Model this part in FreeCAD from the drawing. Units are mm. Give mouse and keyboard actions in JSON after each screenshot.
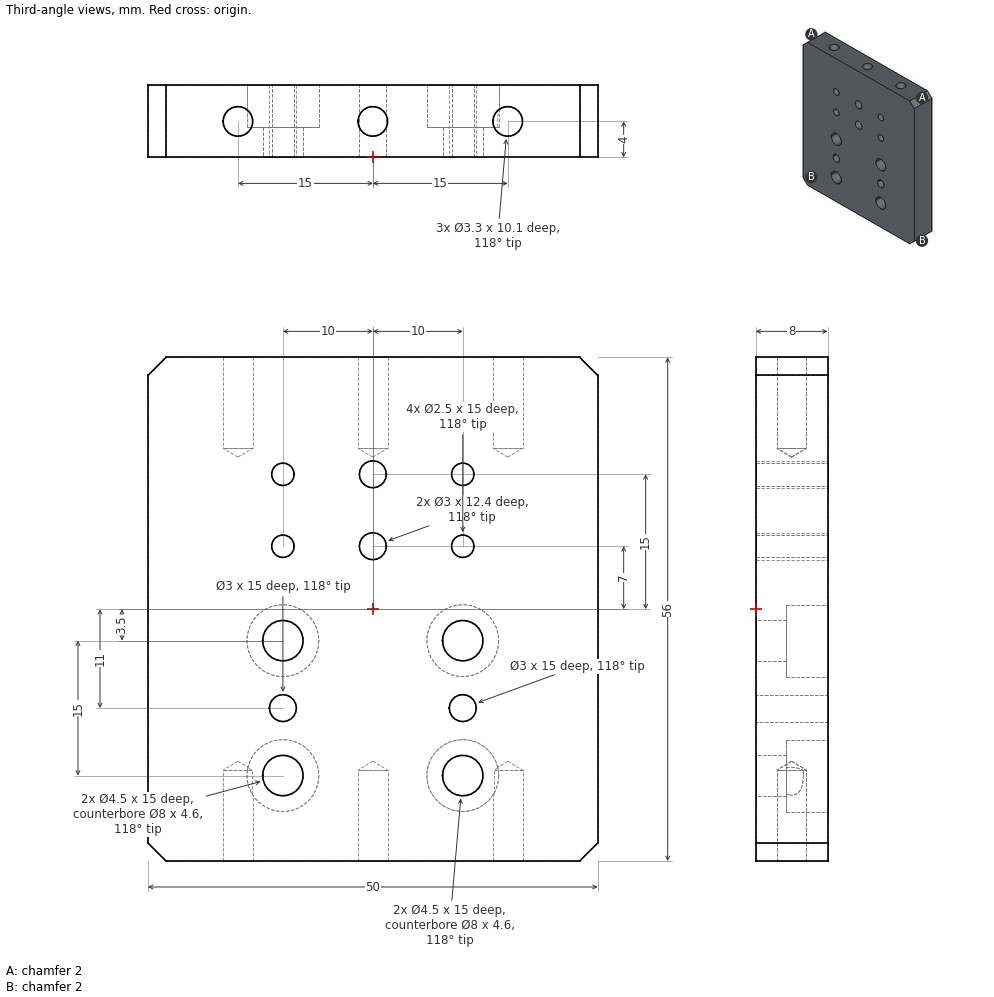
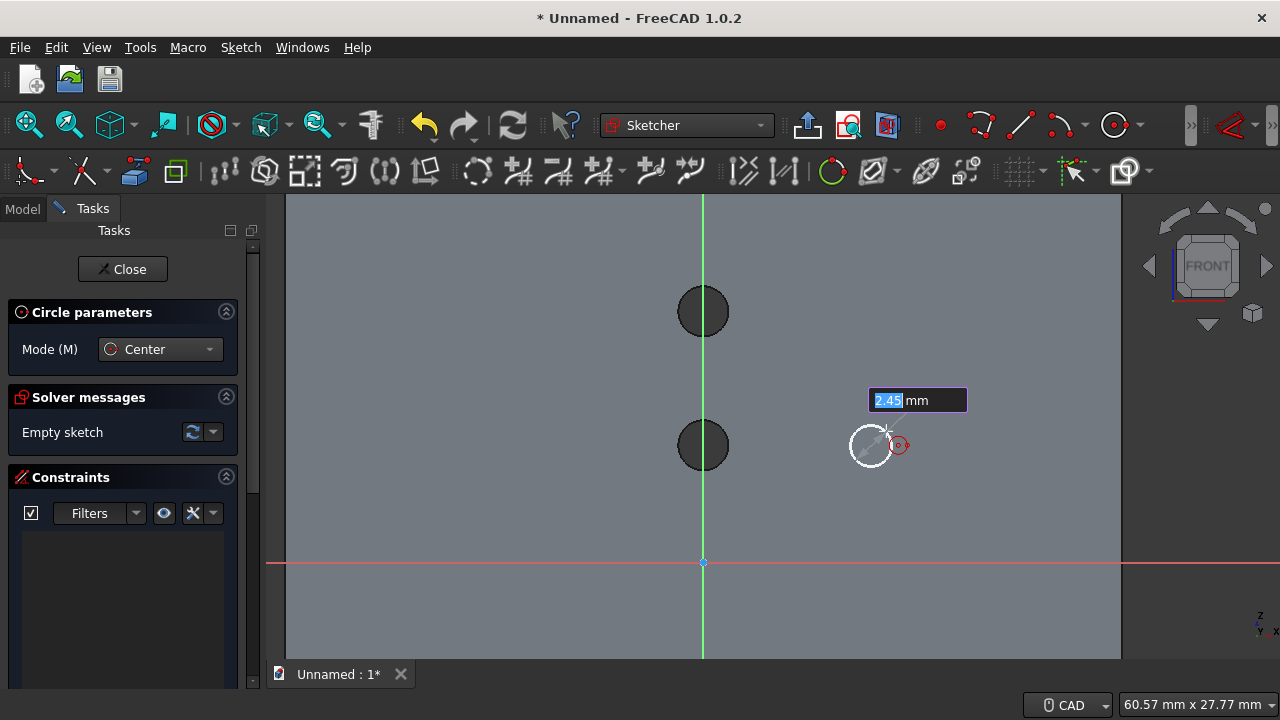
{"action": "type", "text": "2.5"}
{"action": "key", "text": "Return"}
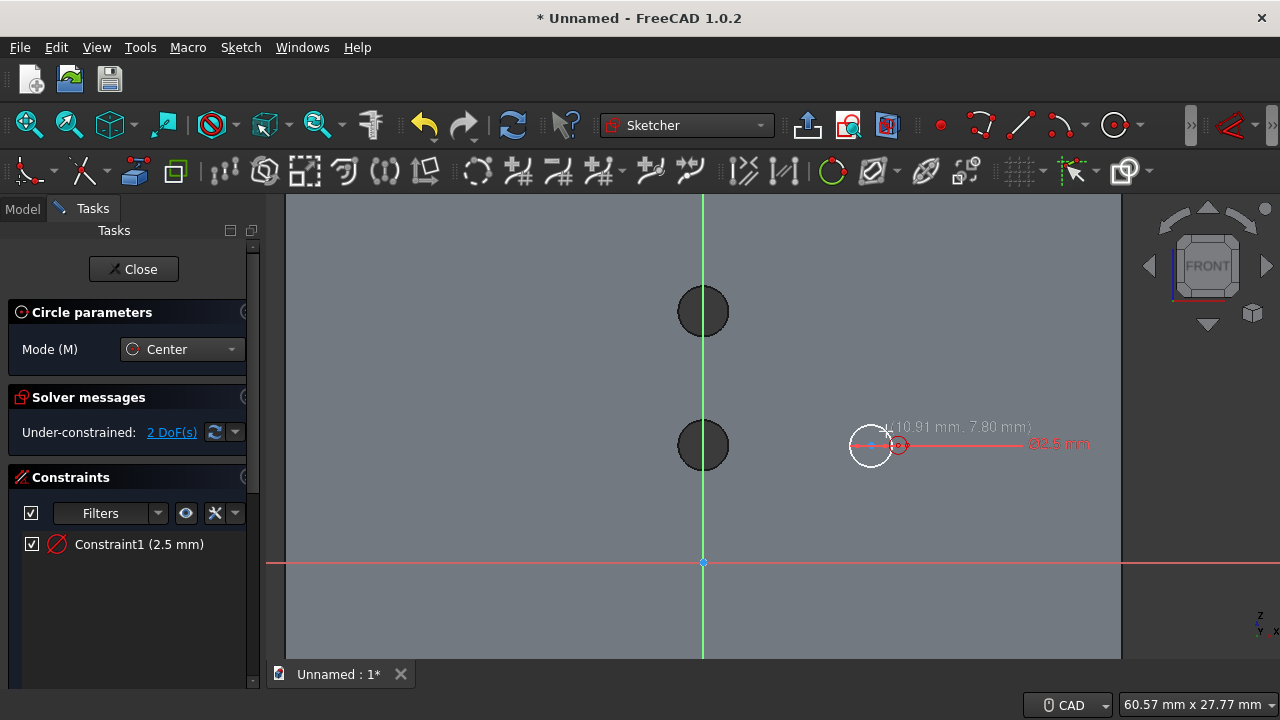
{"action": "left_click", "coordinate": [536, 445]}
{"action": "mouse_move", "coordinate": [551, 431]}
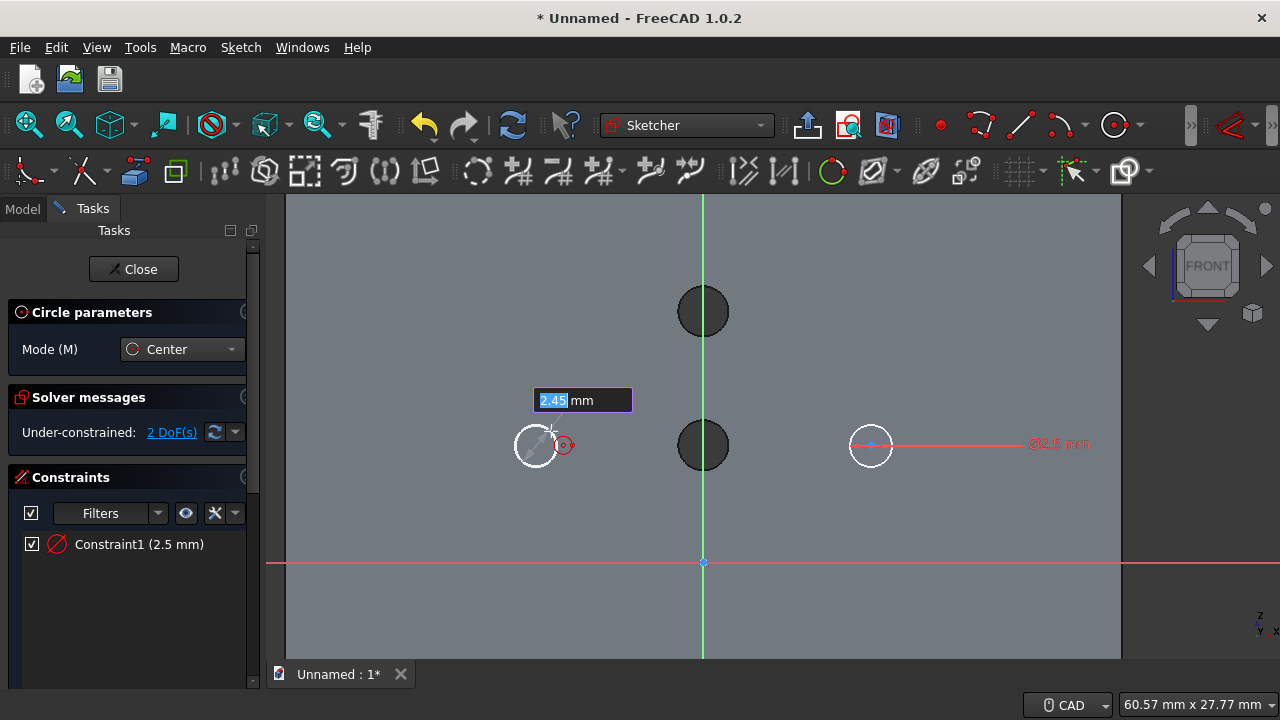
{"action": "type", "text": "2.5"}
{"action": "key", "text": "Return"}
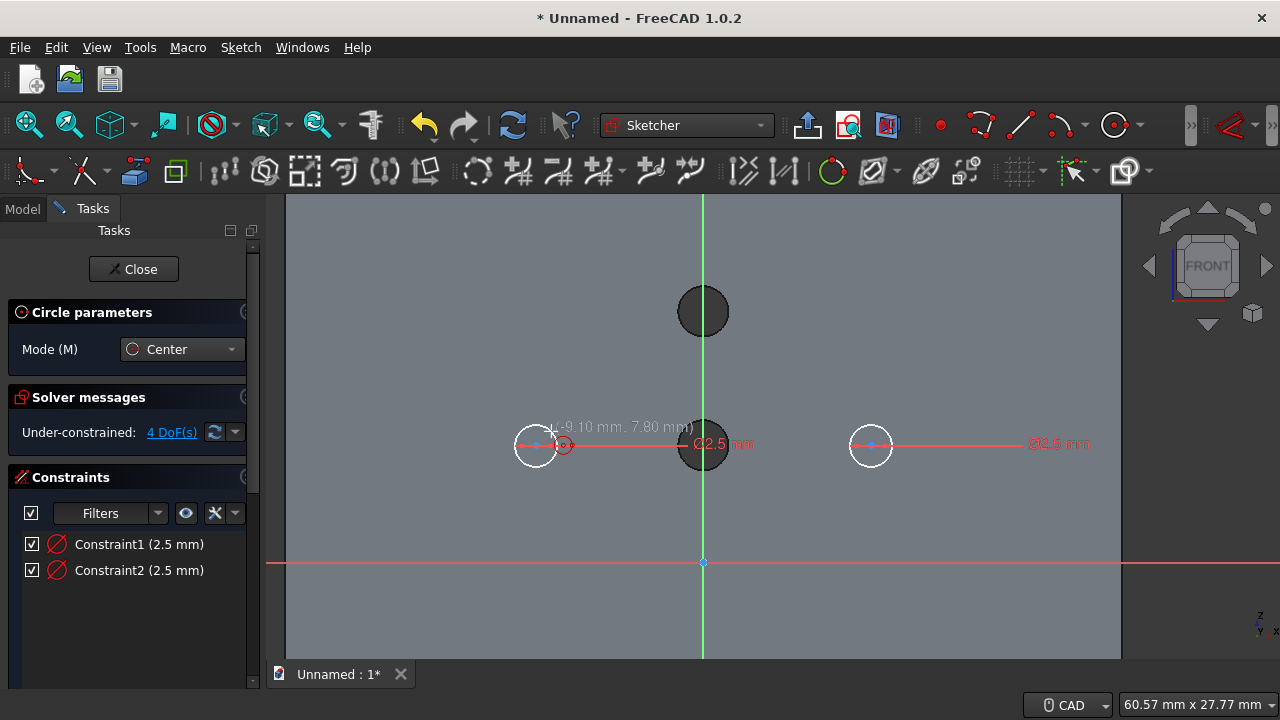
{"action": "left_click", "coordinate": [871, 311]}
{"action": "mouse_move", "coordinate": [886, 297]}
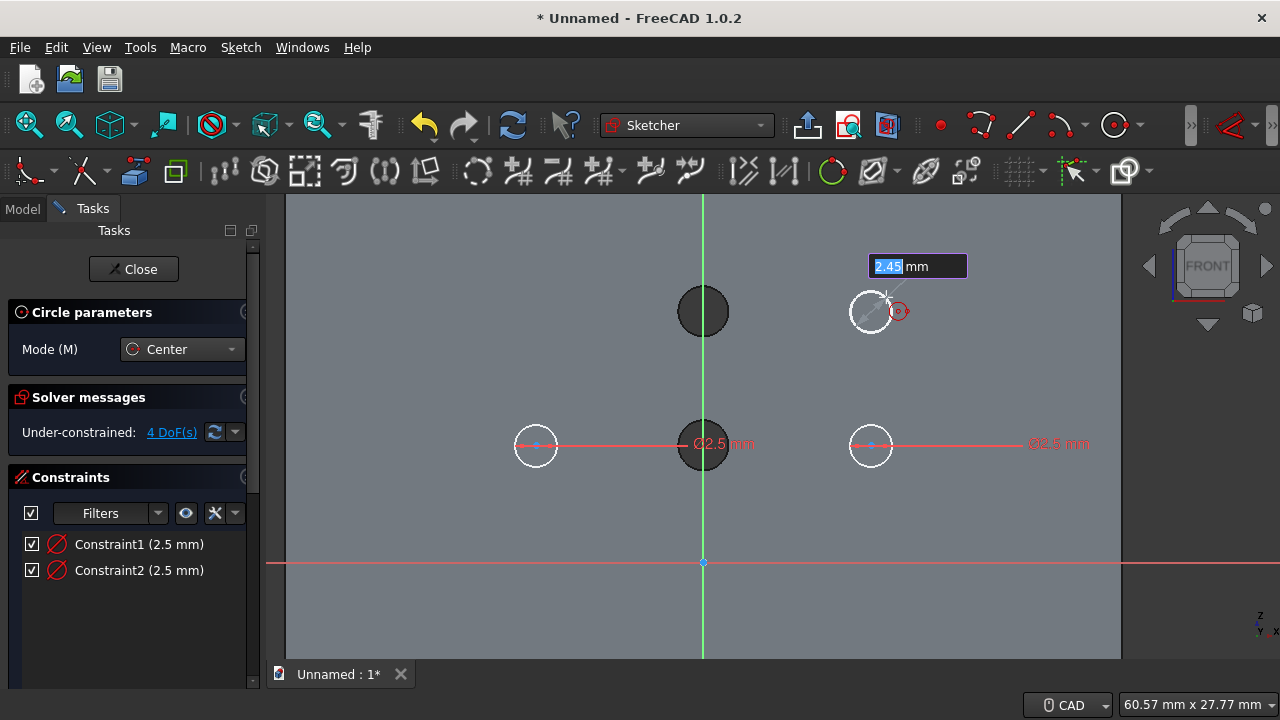
{"action": "type", "text": "2.5"}
{"action": "key", "text": "Return"}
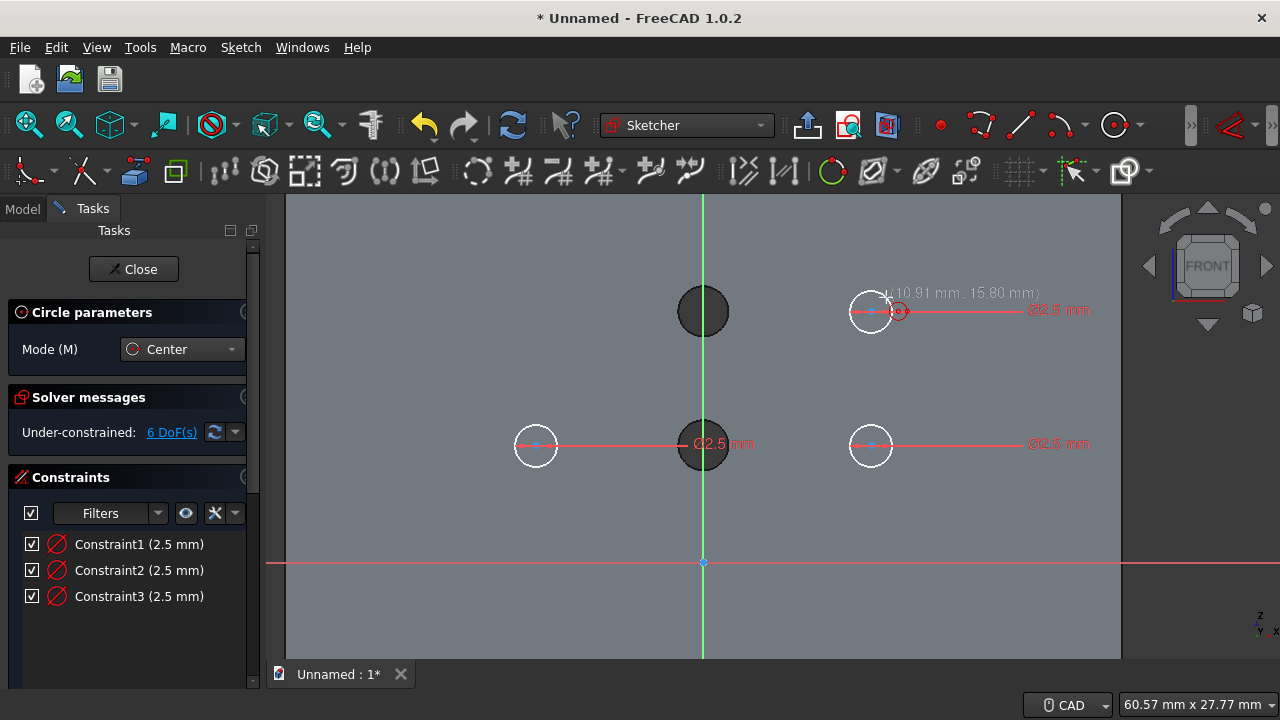
{"action": "left_click", "coordinate": [536, 311]}
{"action": "mouse_move", "coordinate": [551, 297]}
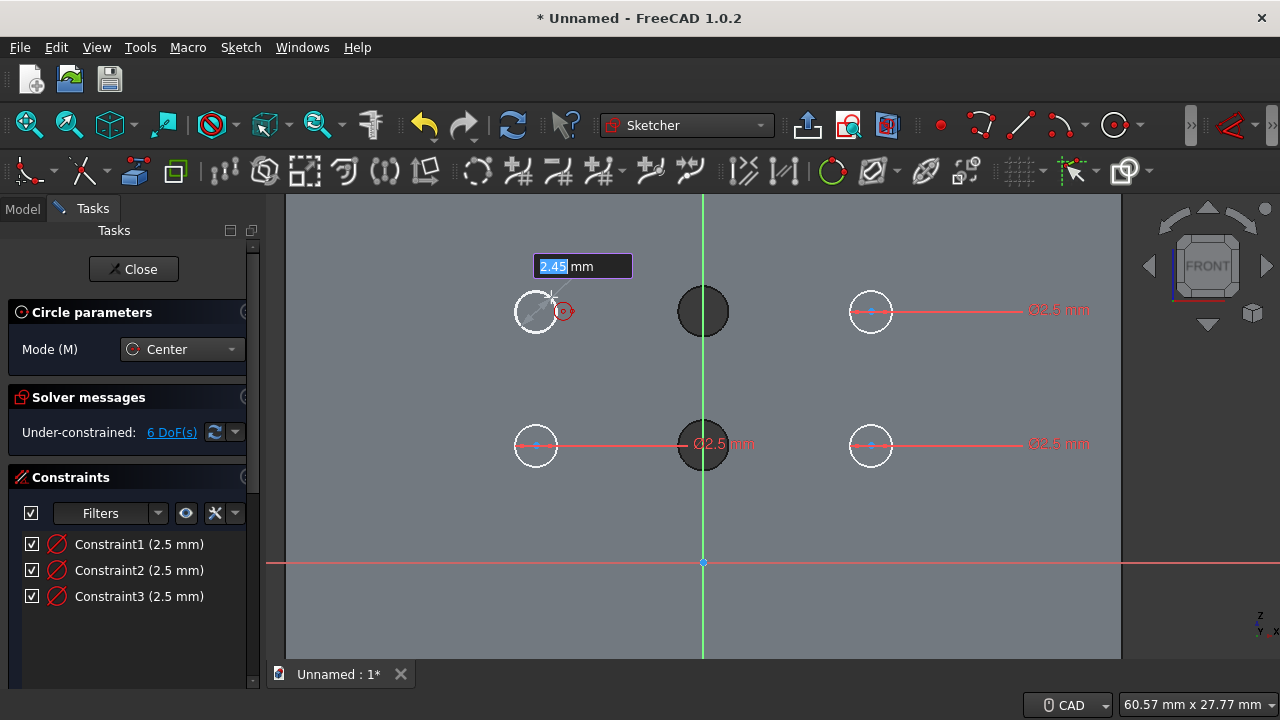
{"action": "type", "text": "2.5"}
{"action": "key", "text": "Return"}
{"action": "key", "text": "Escape"}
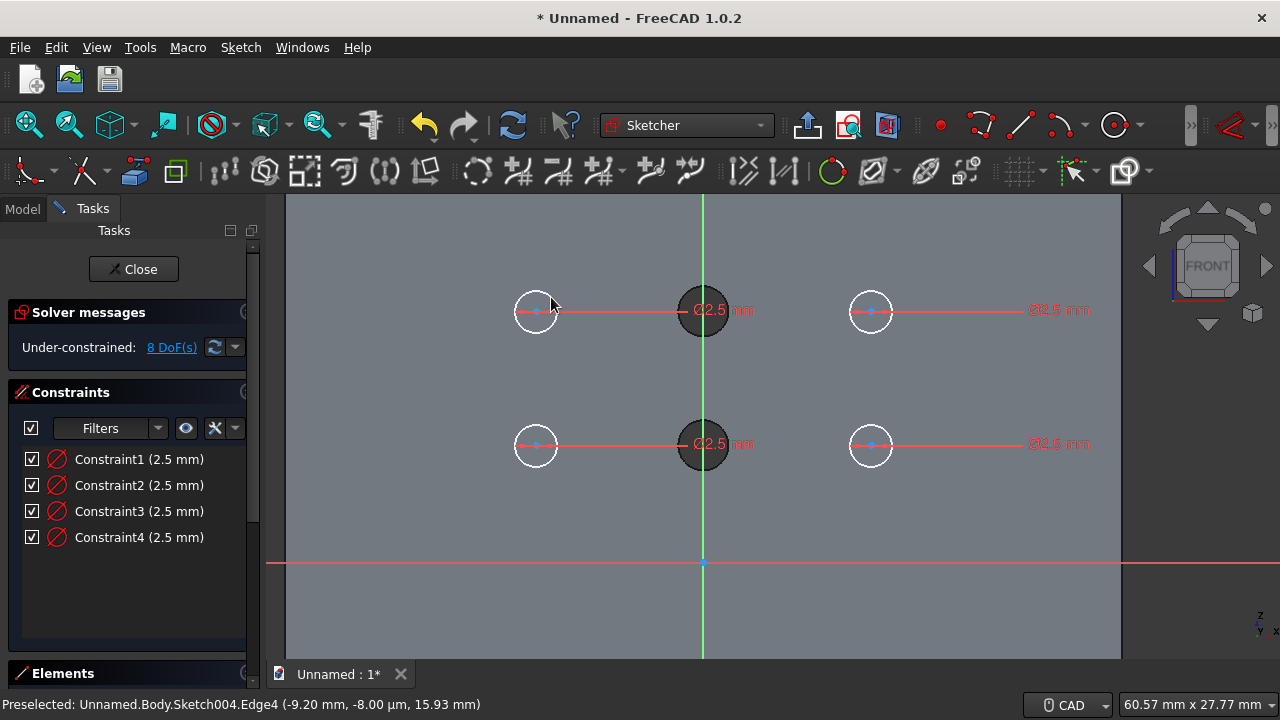
{"action": "left_click", "coordinate": [871, 446]}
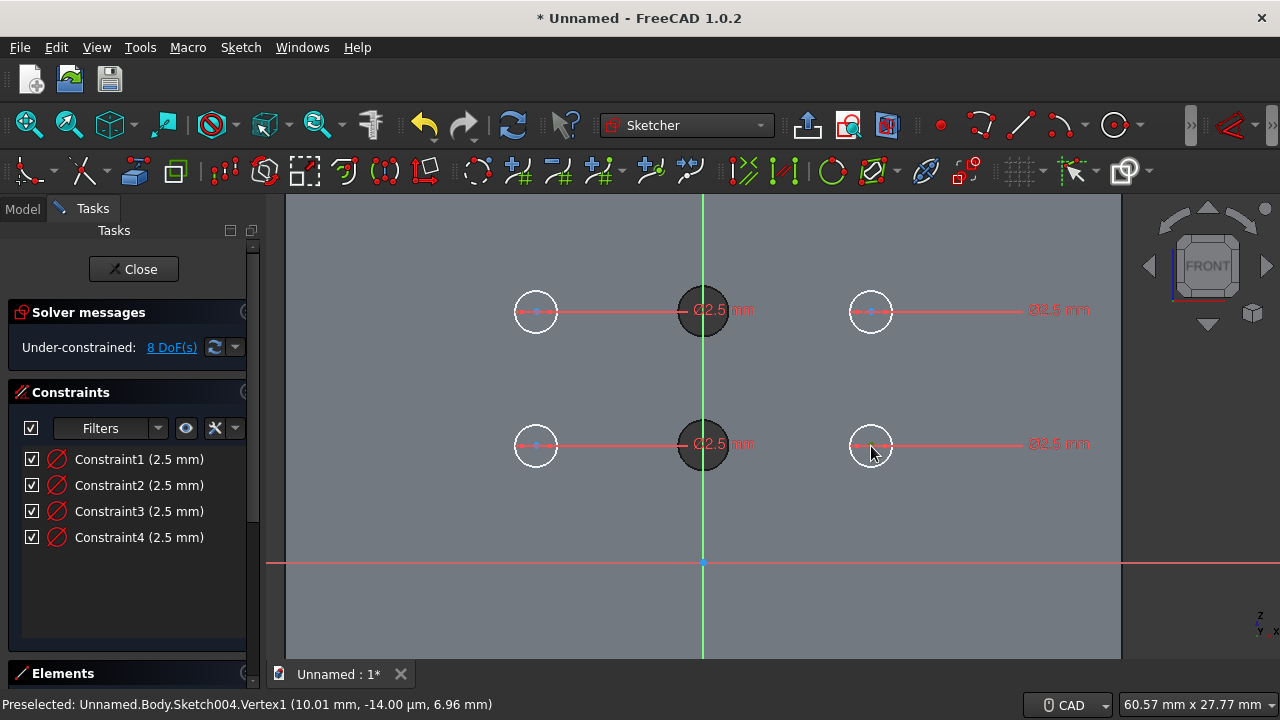
{"action": "left_click", "coordinate": [536, 446]}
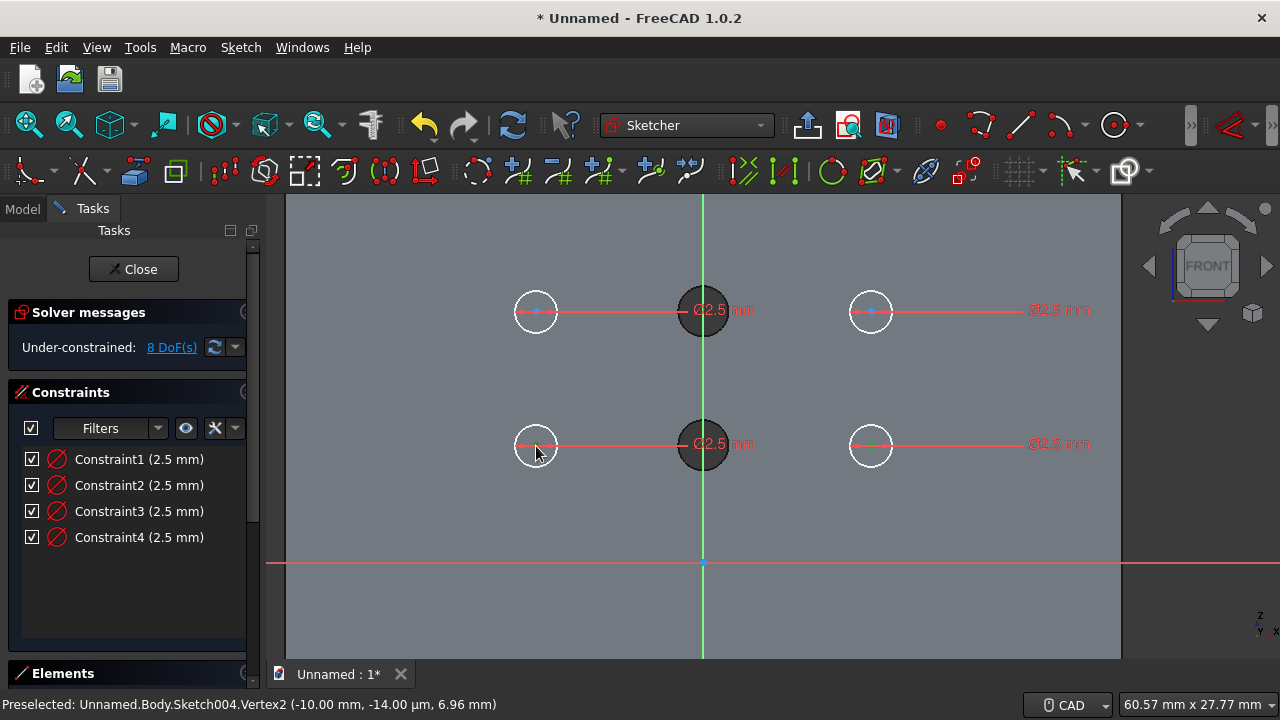
{"action": "key", "text": "h"}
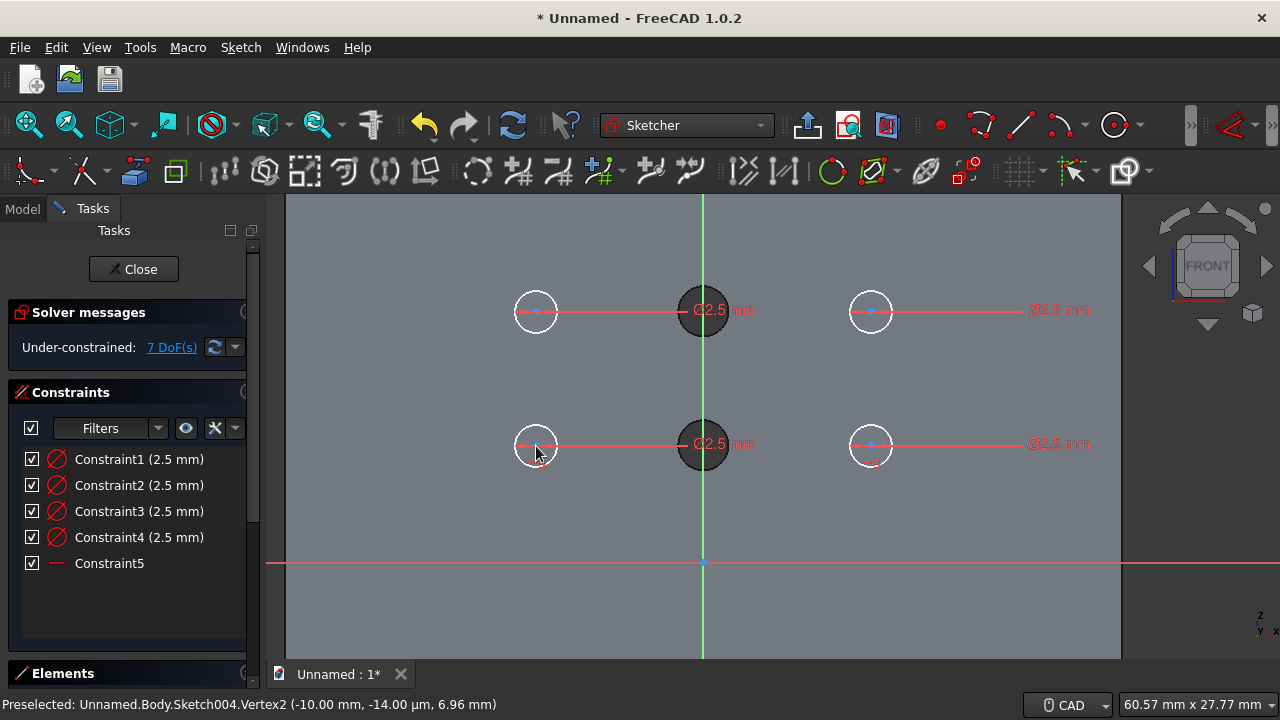
{"action": "left_click", "coordinate": [871, 446]}